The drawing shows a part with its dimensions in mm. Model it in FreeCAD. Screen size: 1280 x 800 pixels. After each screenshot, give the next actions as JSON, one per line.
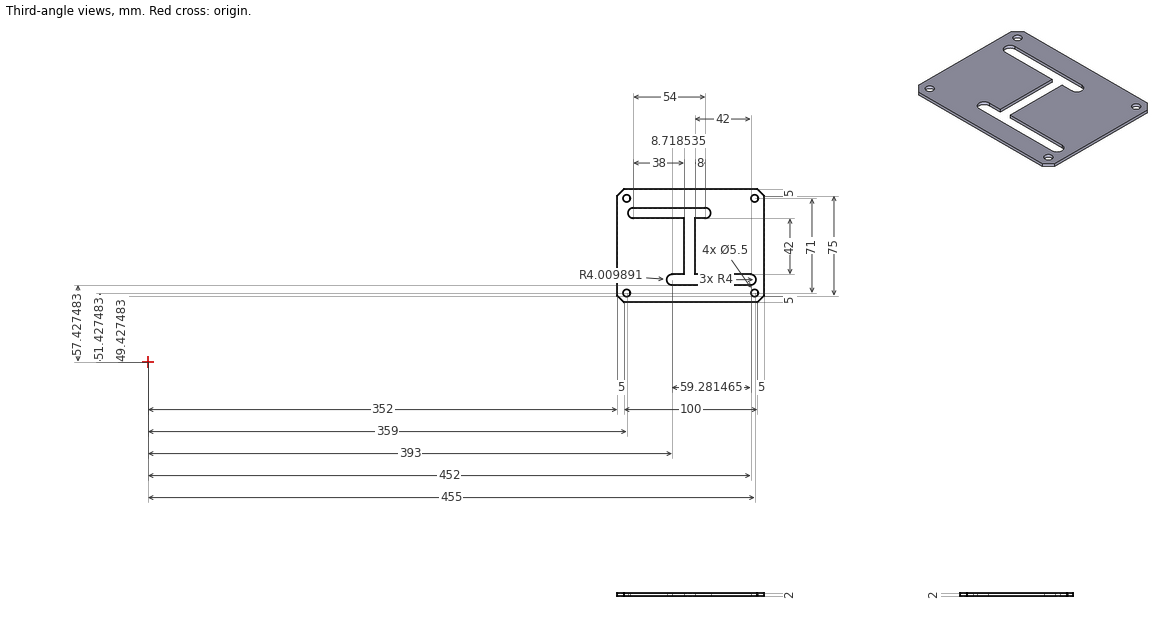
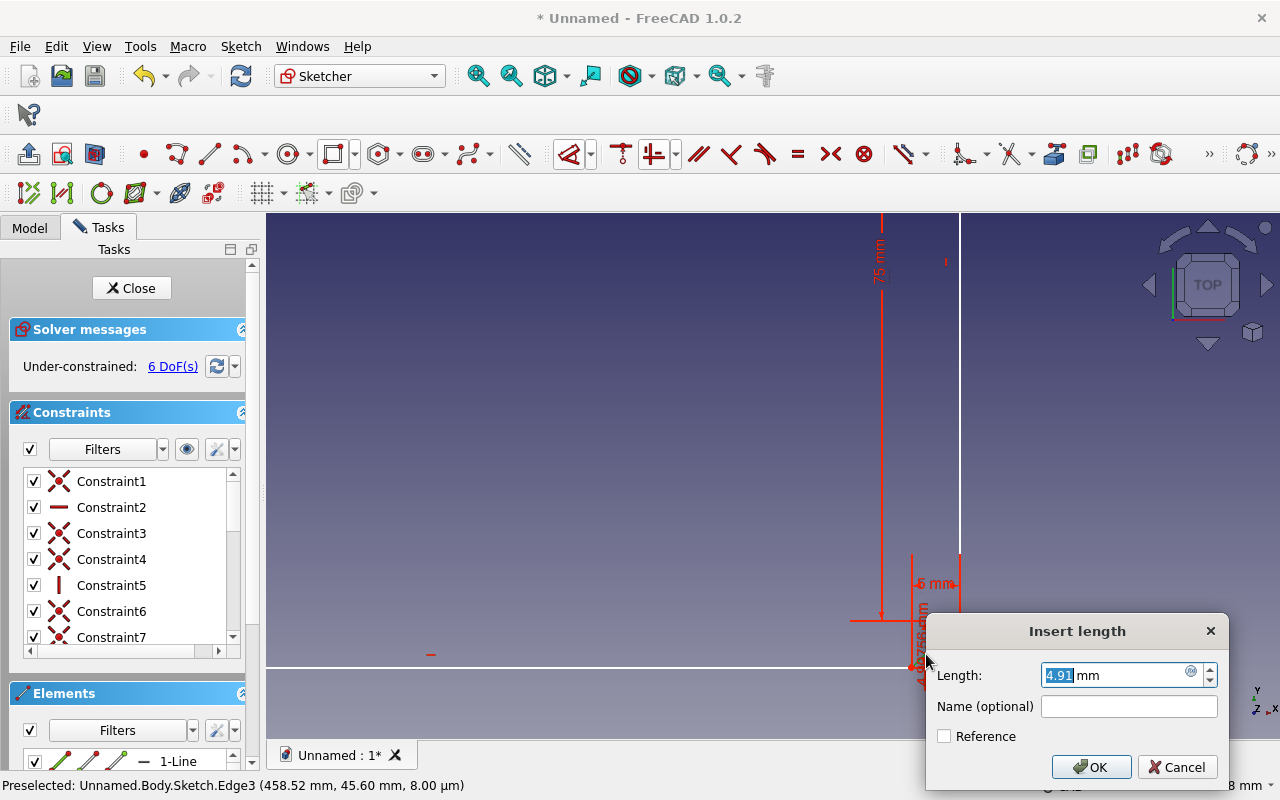
{"action": "type", "text": "5"}
{"action": "key", "text": "Return"}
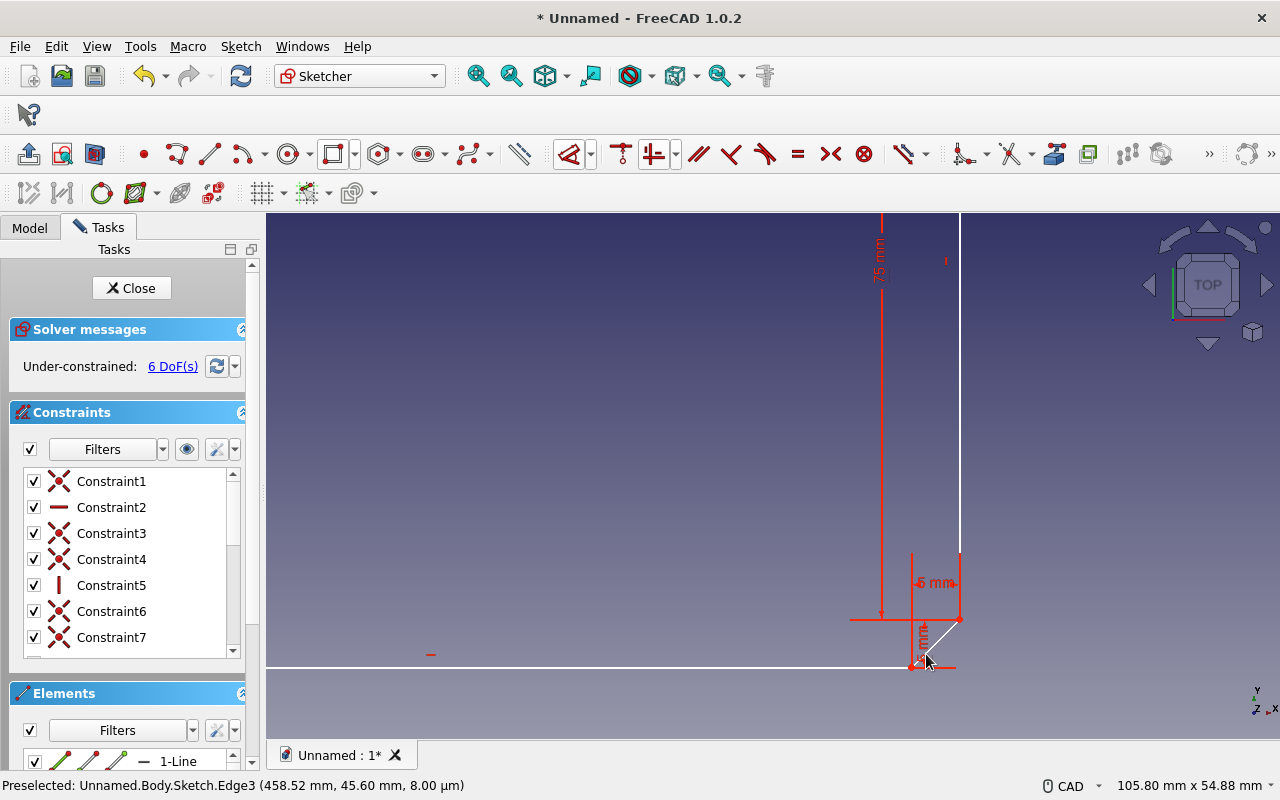
{"action": "scroll", "coordinate": [927, 654], "scroll_direction": "down", "scroll_amount": 4}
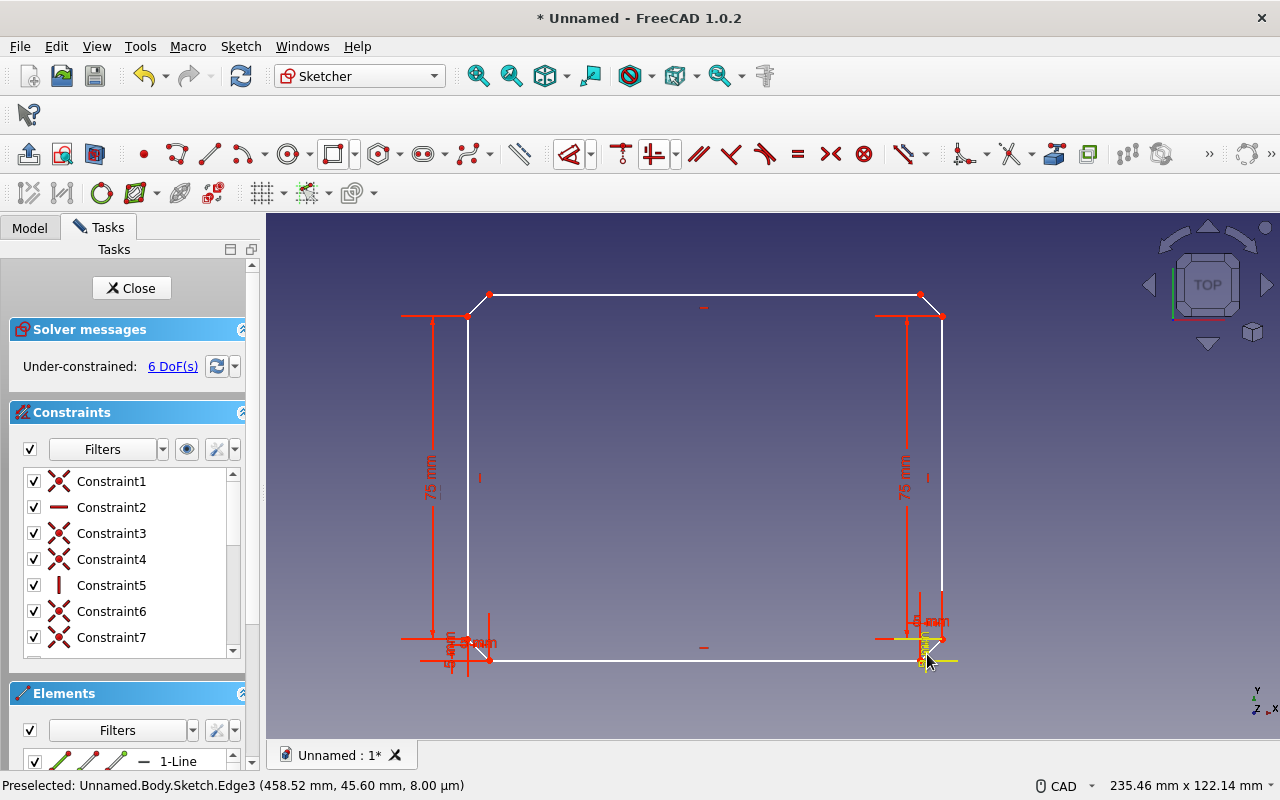
{"action": "scroll", "coordinate": [935, 310], "scroll_direction": "up", "scroll_amount": 4}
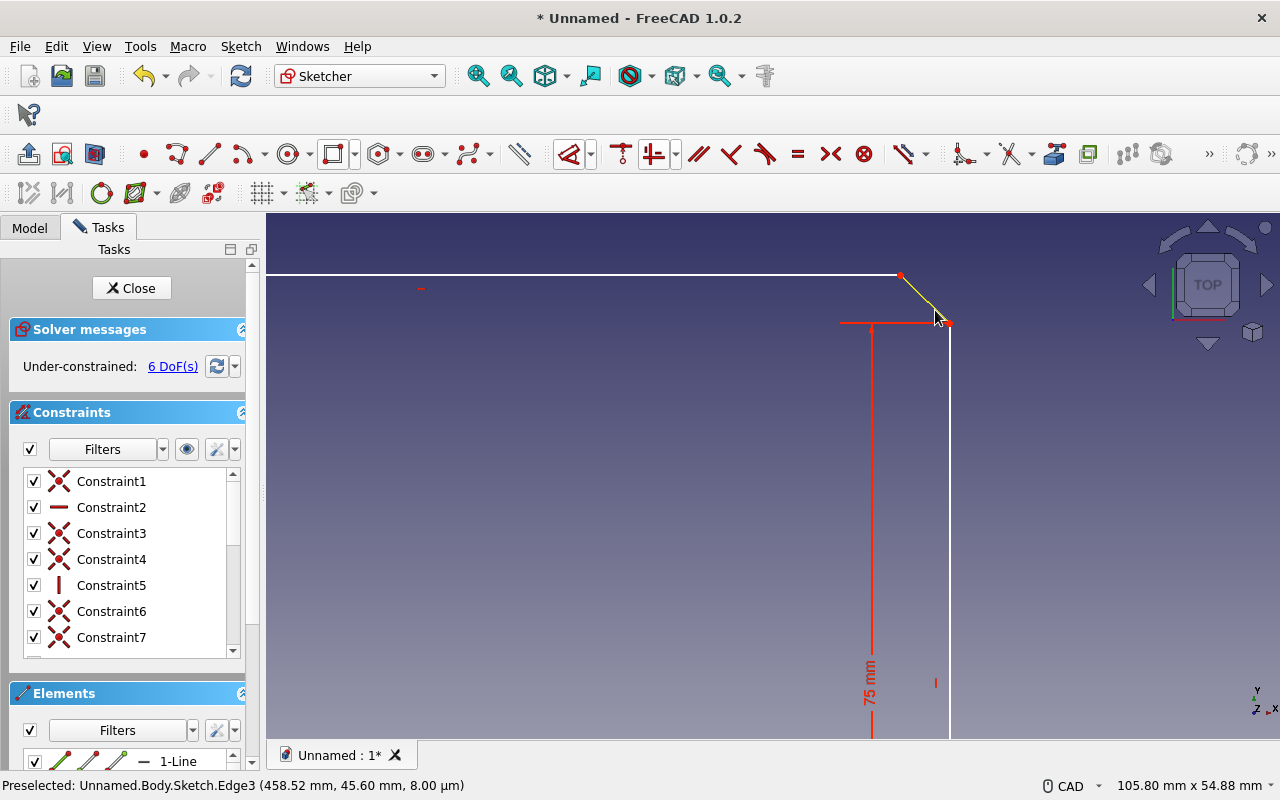
{"action": "left_click", "coordinate": [935, 309]}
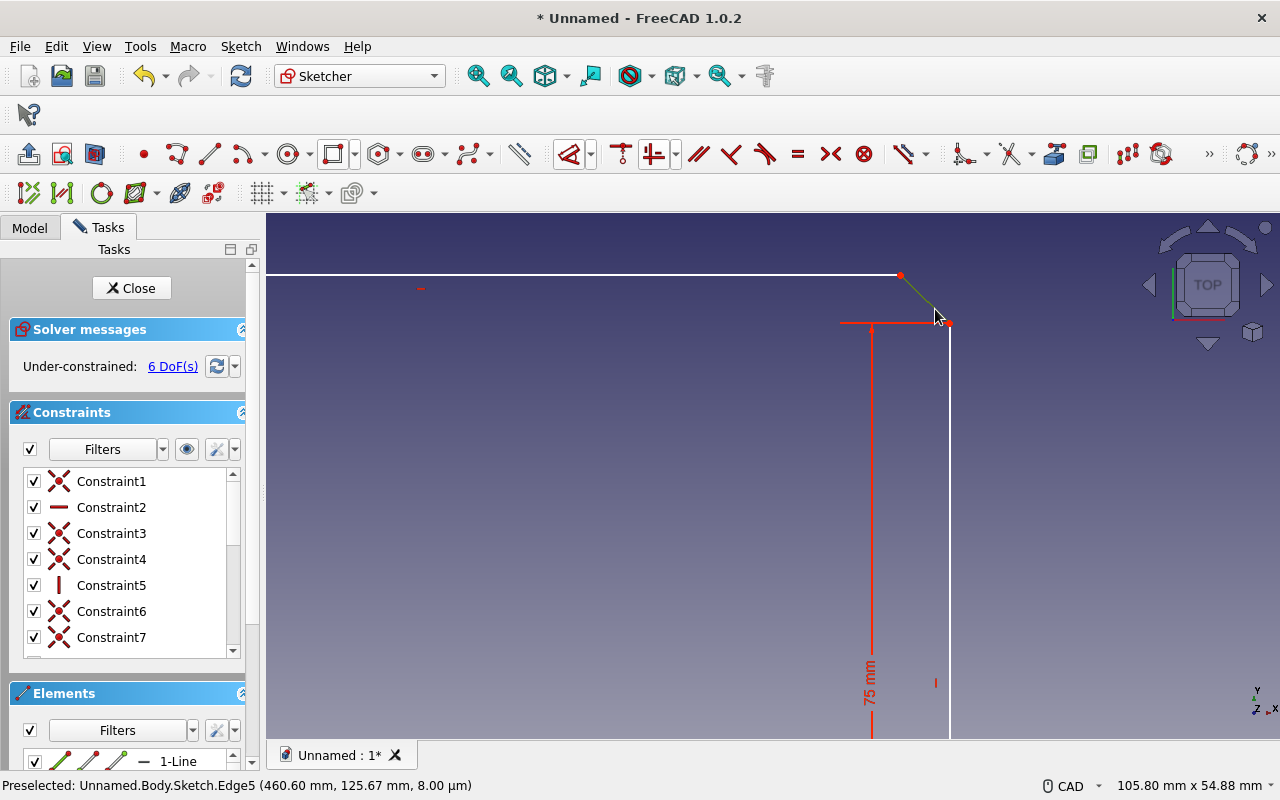
{"action": "left_click", "coordinate": [590, 154]}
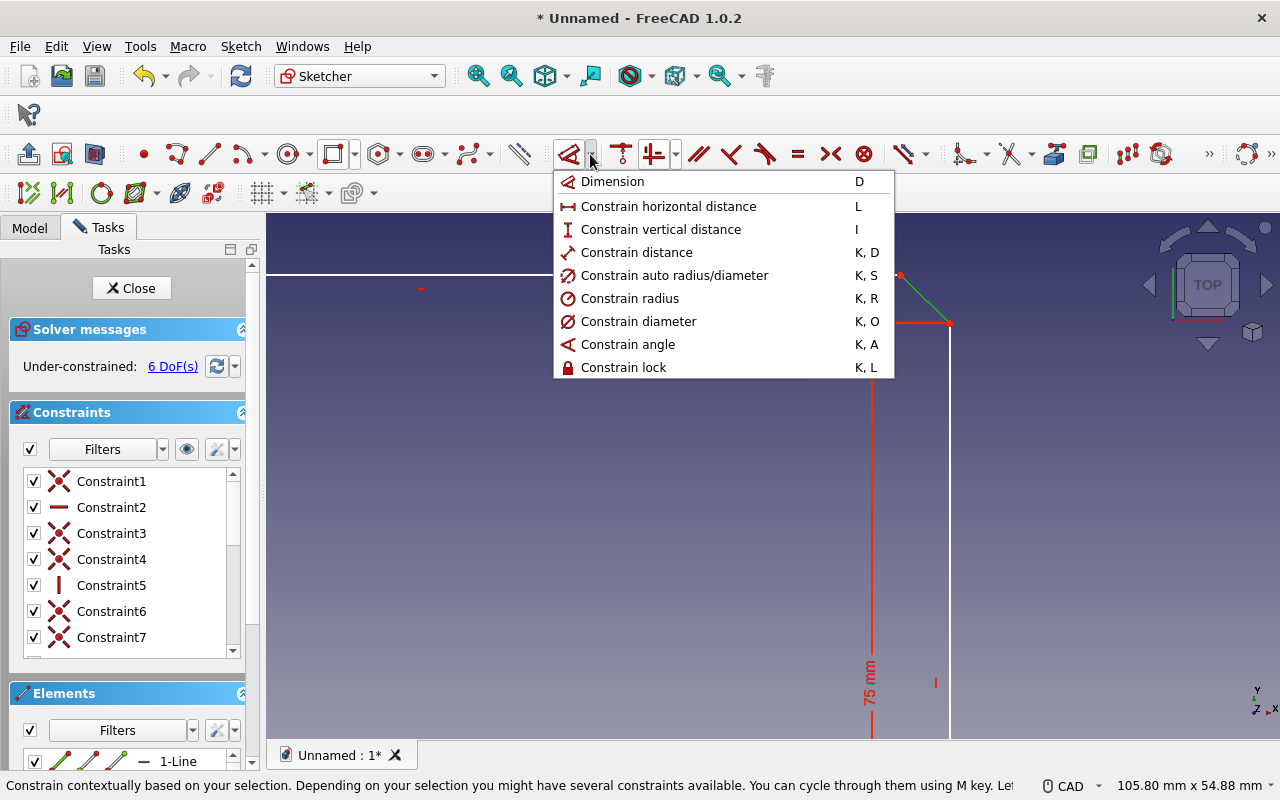
{"action": "left_click", "coordinate": [724, 206]}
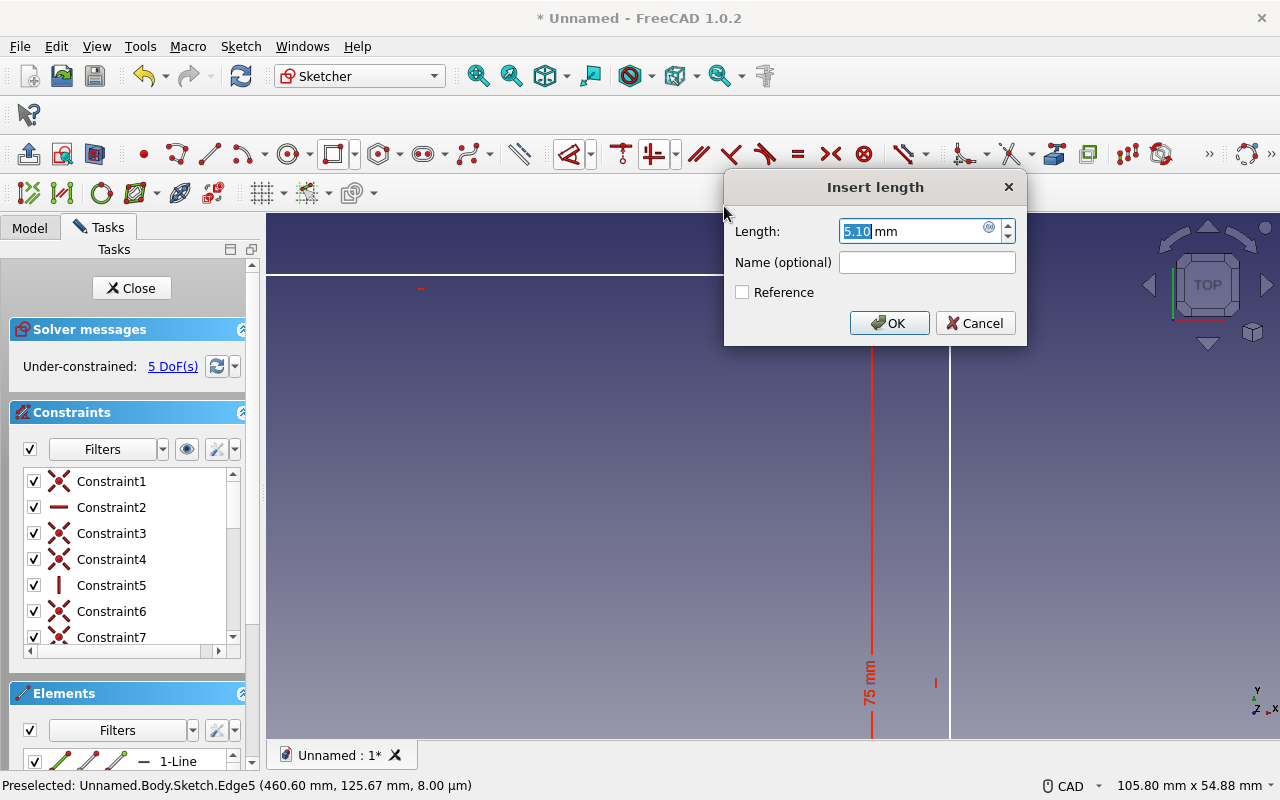
{"action": "type", "text": "5"}
{"action": "key", "text": "Return"}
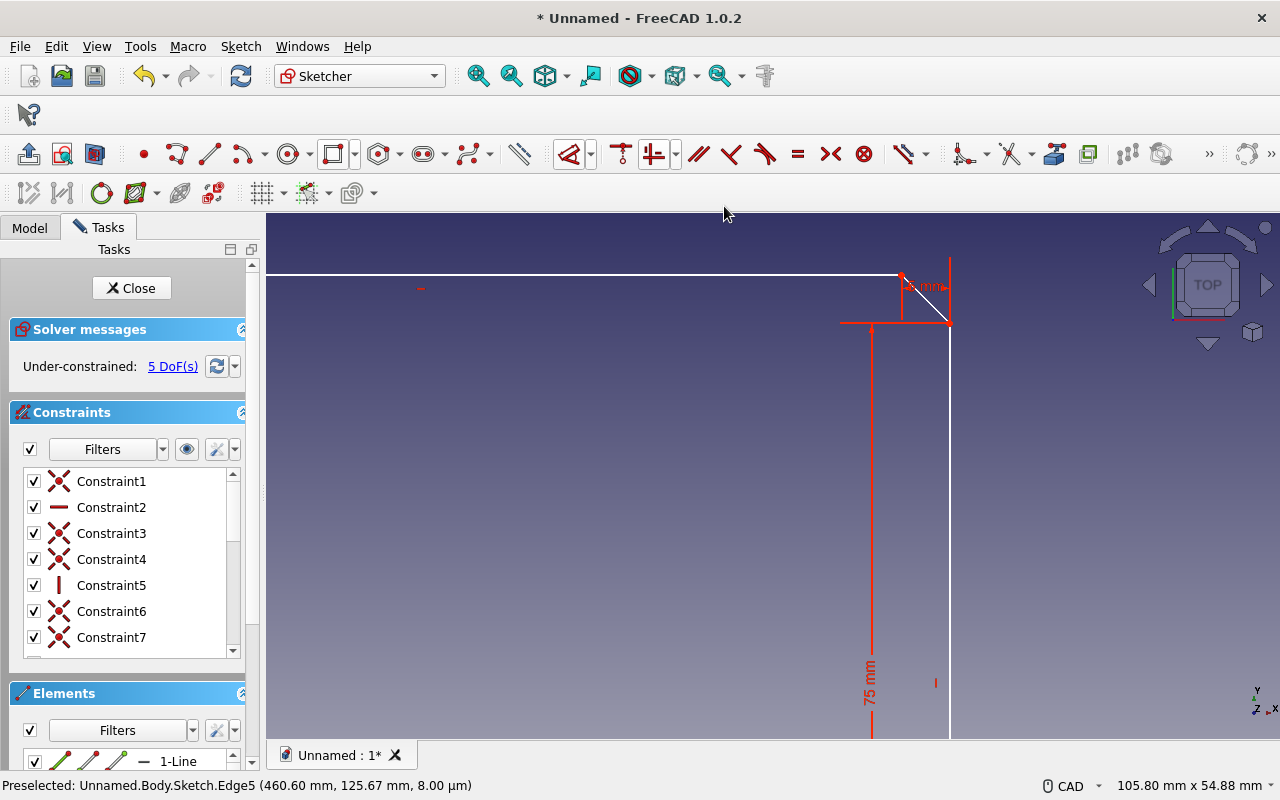
{"action": "left_click", "coordinate": [935, 309]}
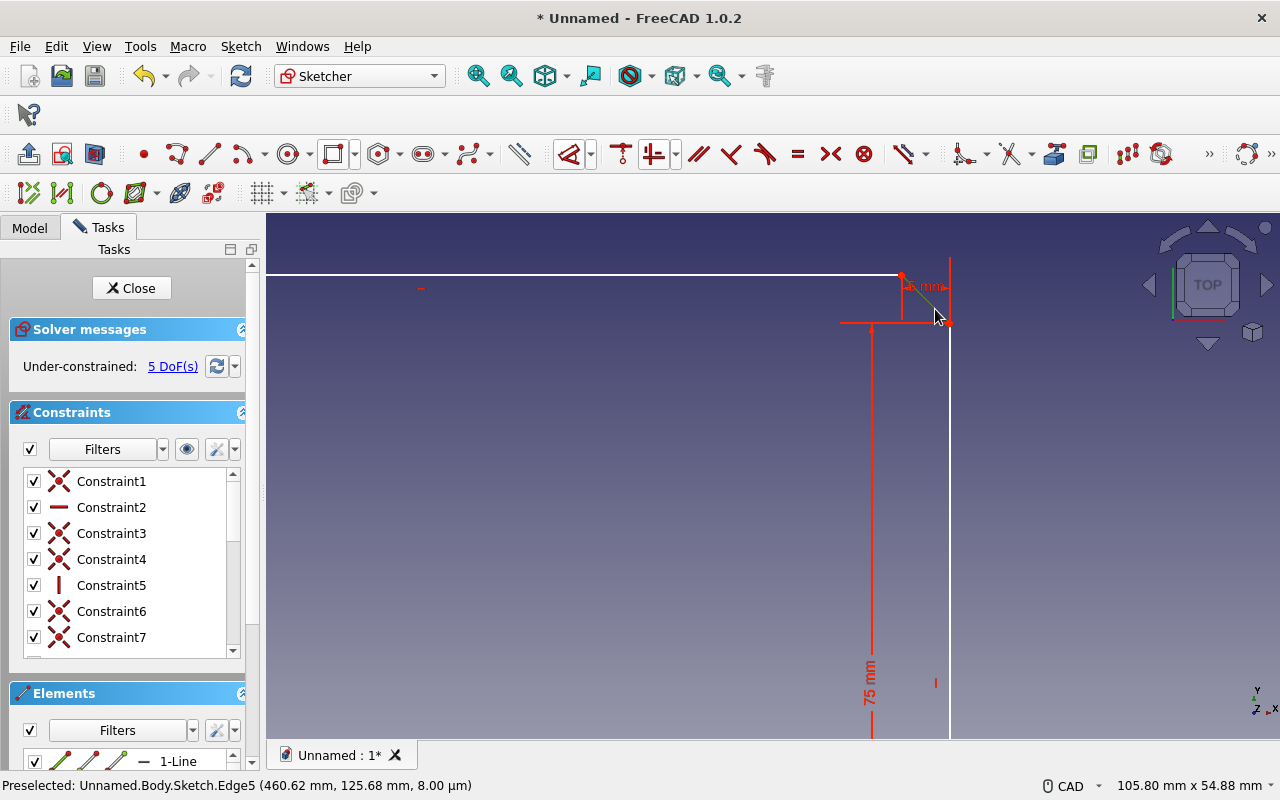
{"action": "key", "text": "i"}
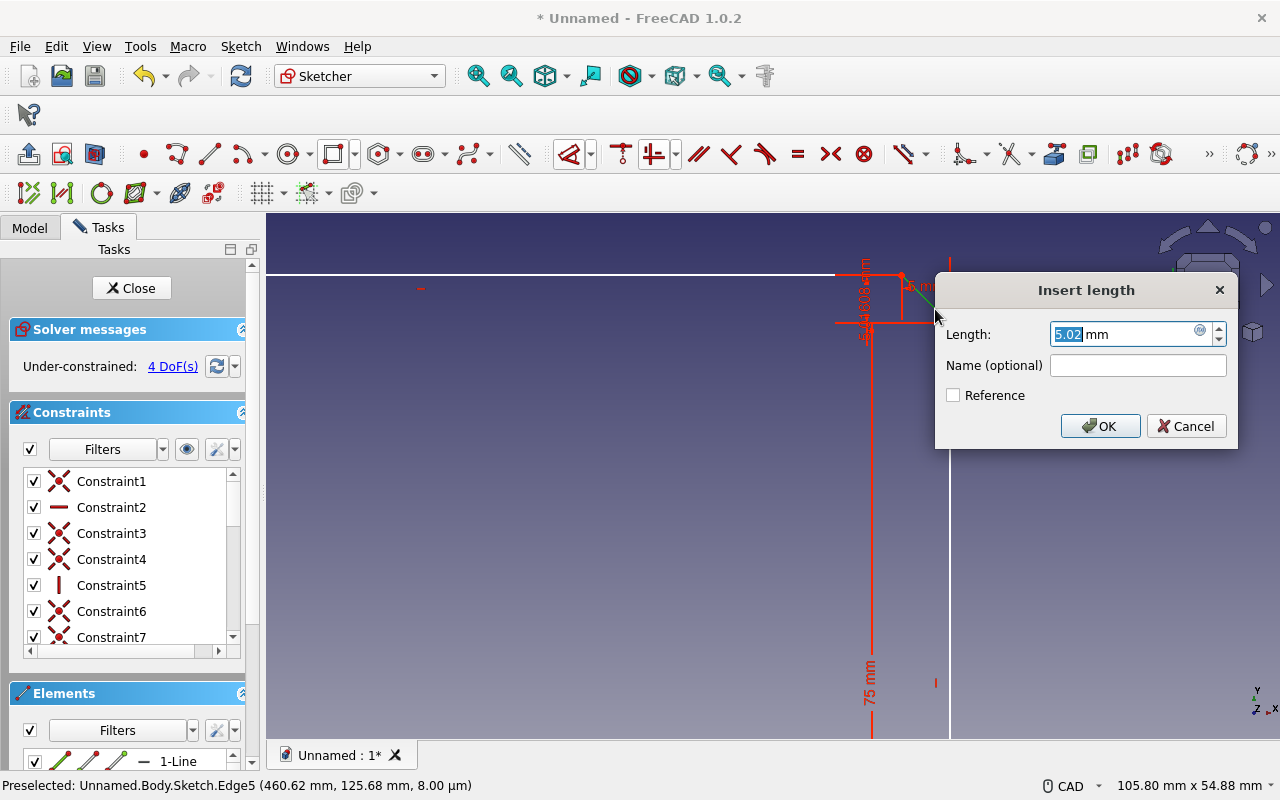
{"action": "type", "text": "5"}
{"action": "key", "text": "Return"}